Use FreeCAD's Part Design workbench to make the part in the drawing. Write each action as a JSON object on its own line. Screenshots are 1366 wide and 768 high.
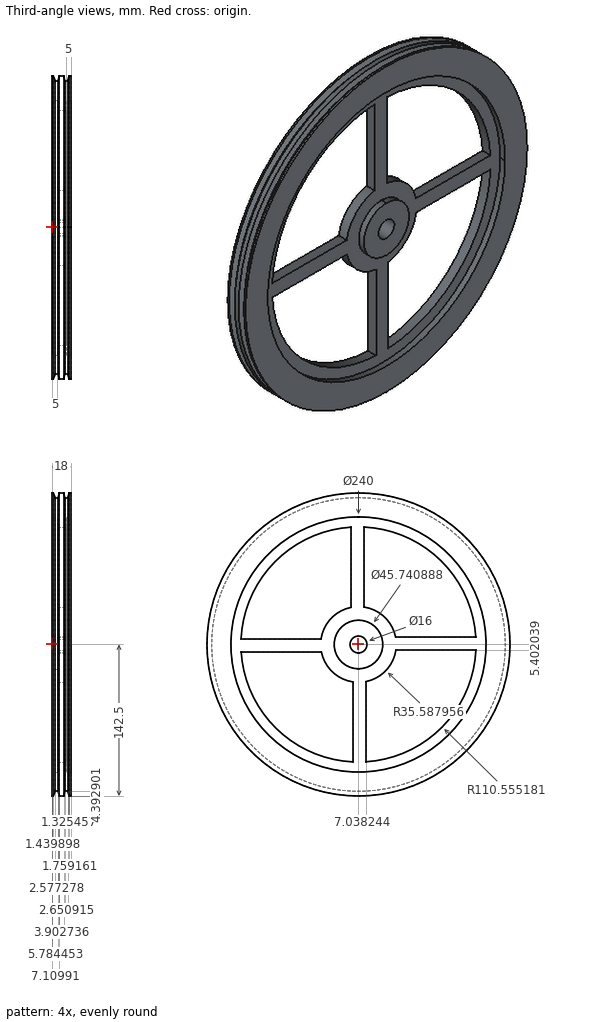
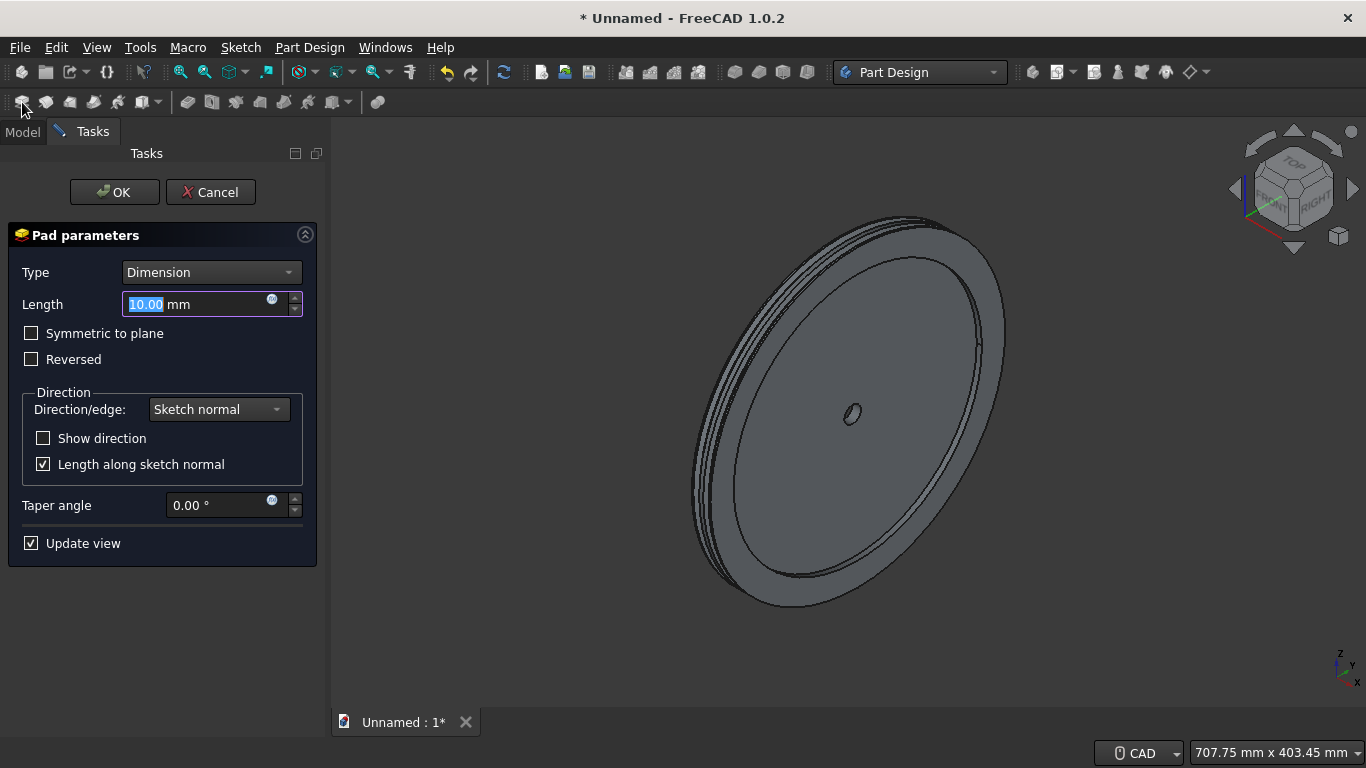
{"action": "type", "text": "5"}
{"action": "key", "text": "Tab"}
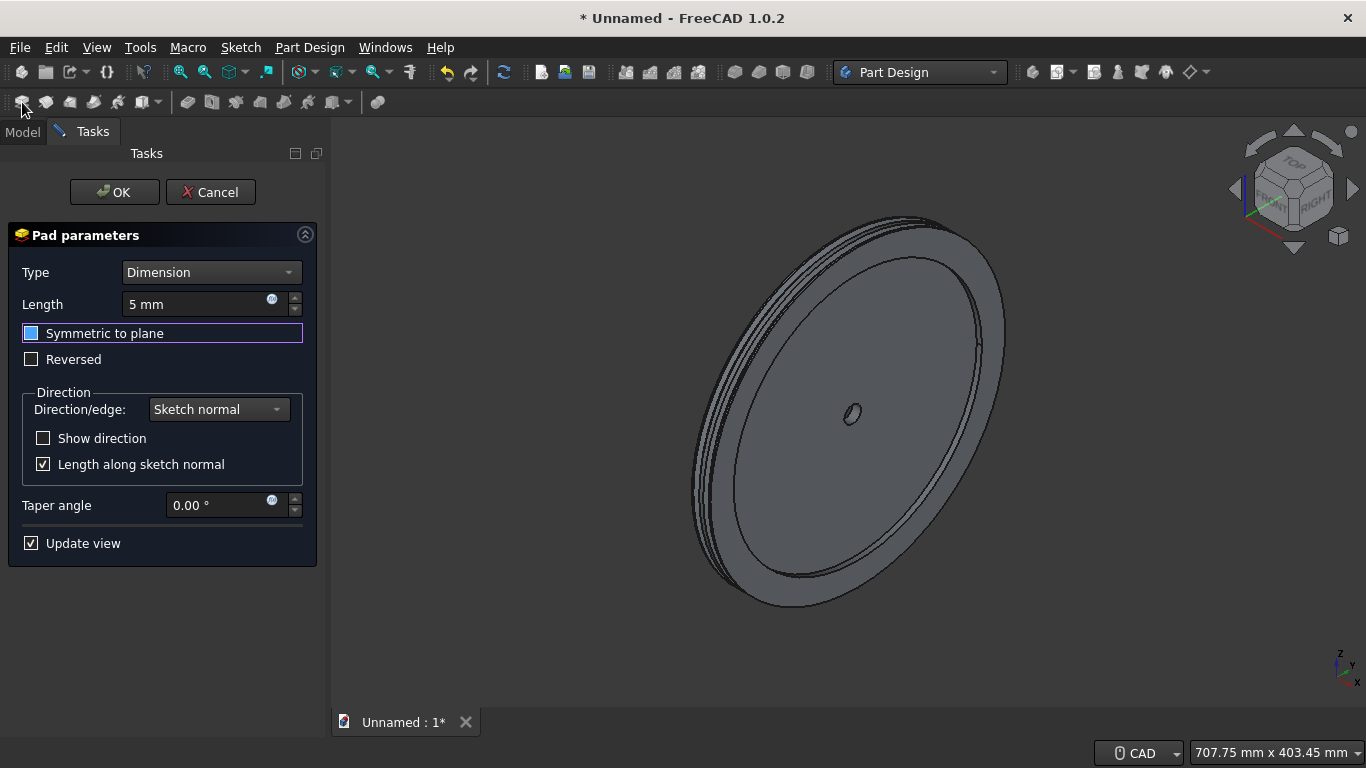
{"action": "left_click", "coordinate": [30, 359]}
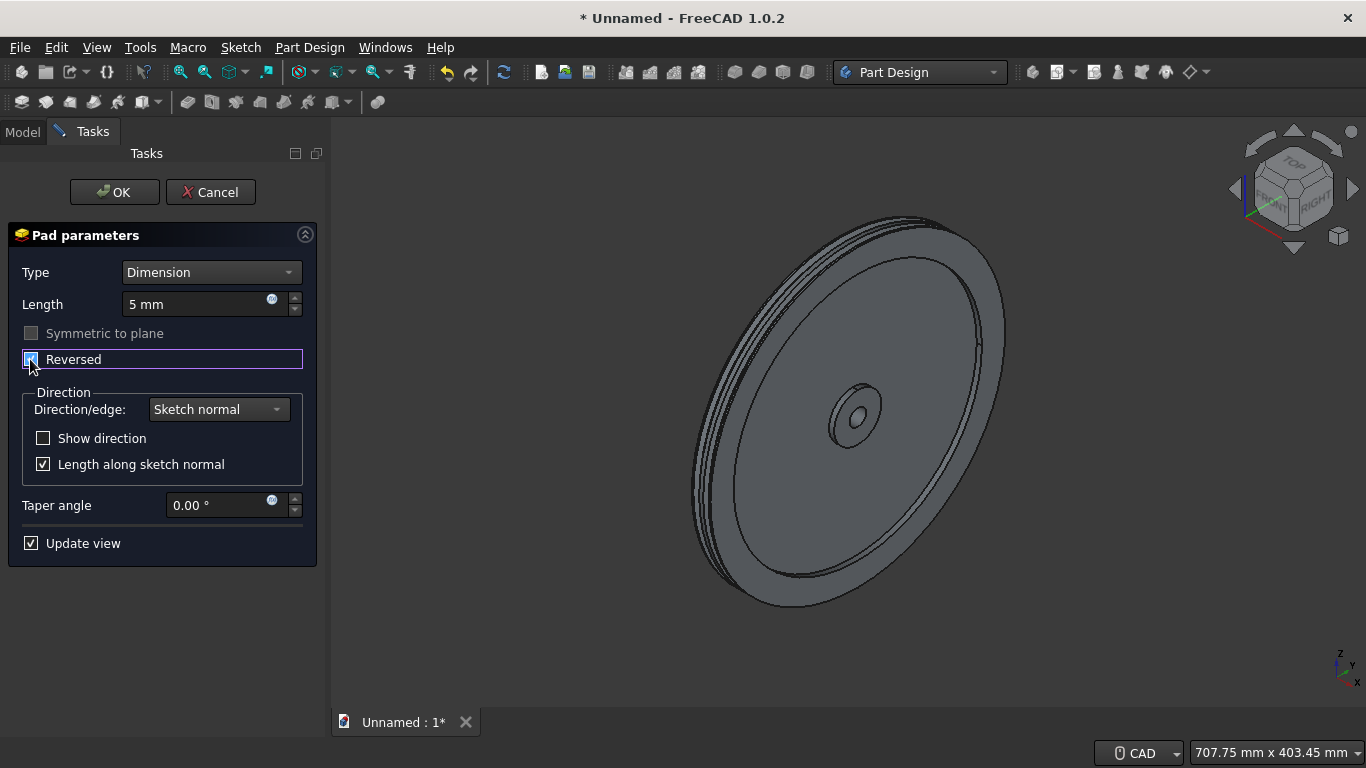
{"action": "left_click", "coordinate": [115, 192]}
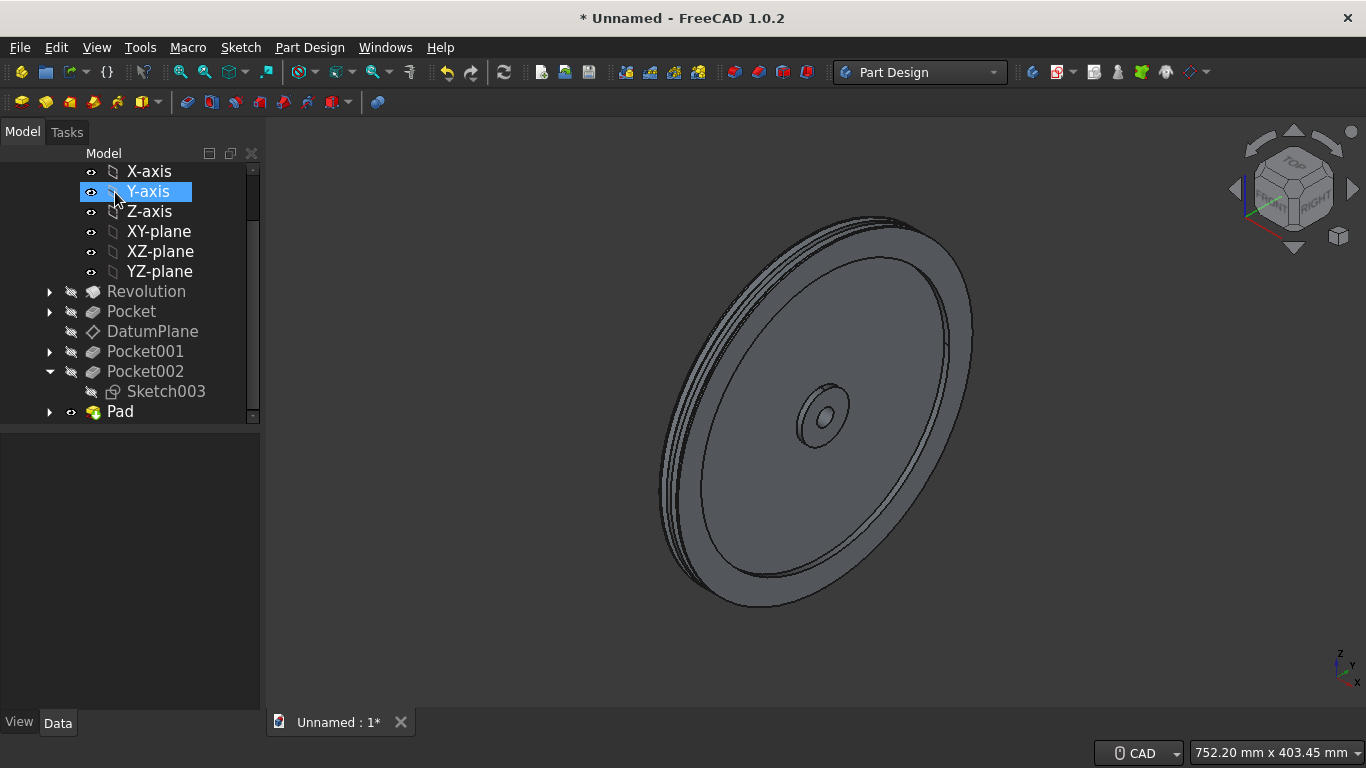
{"action": "key", "text": "6"}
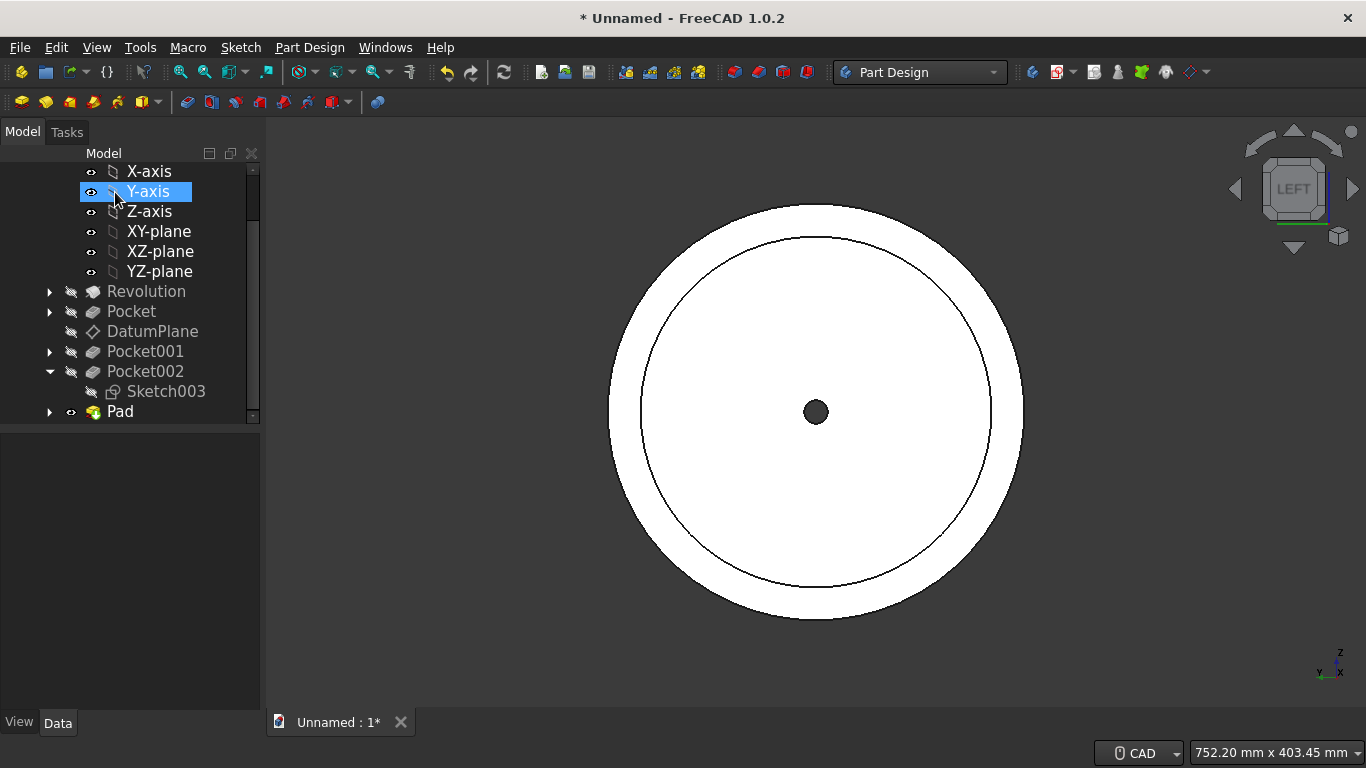
{"action": "left_click", "coordinate": [716, 411]}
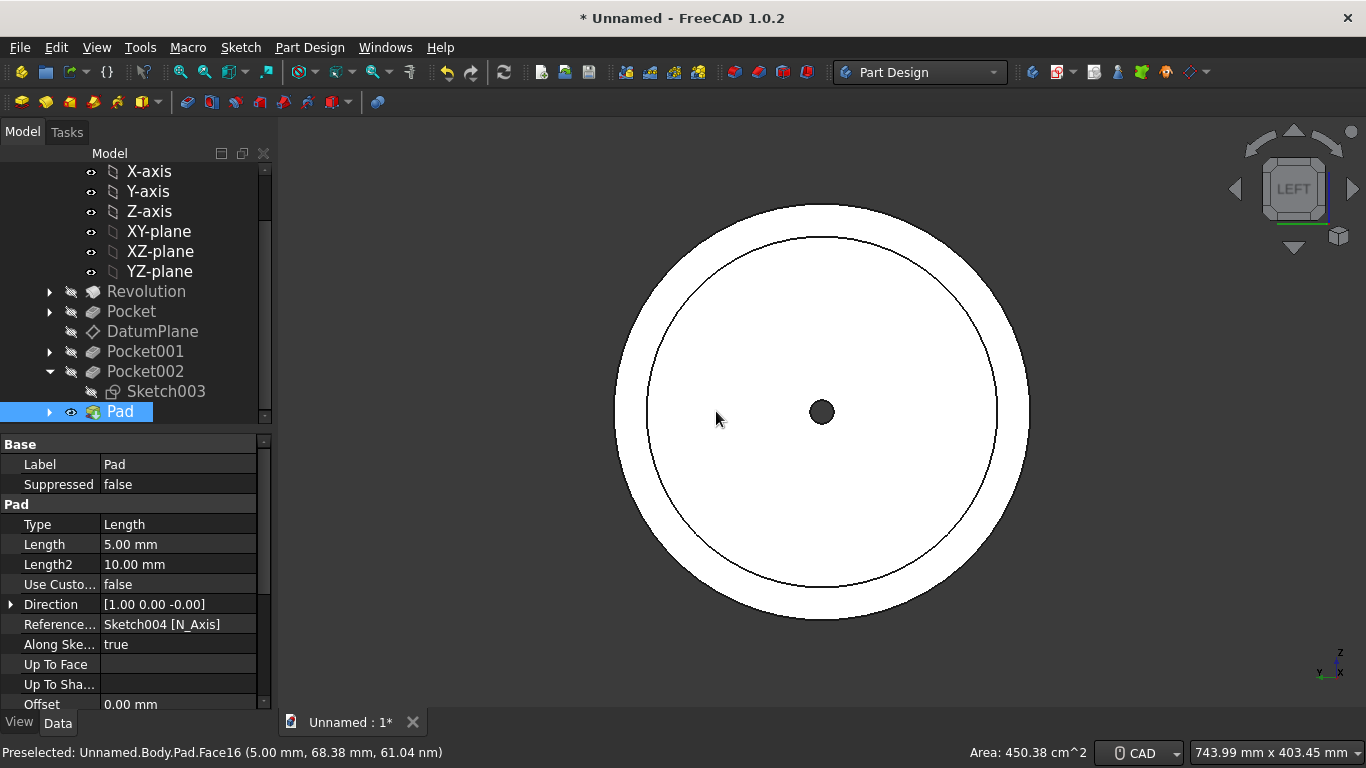
{"action": "left_click", "coordinate": [1058, 72]}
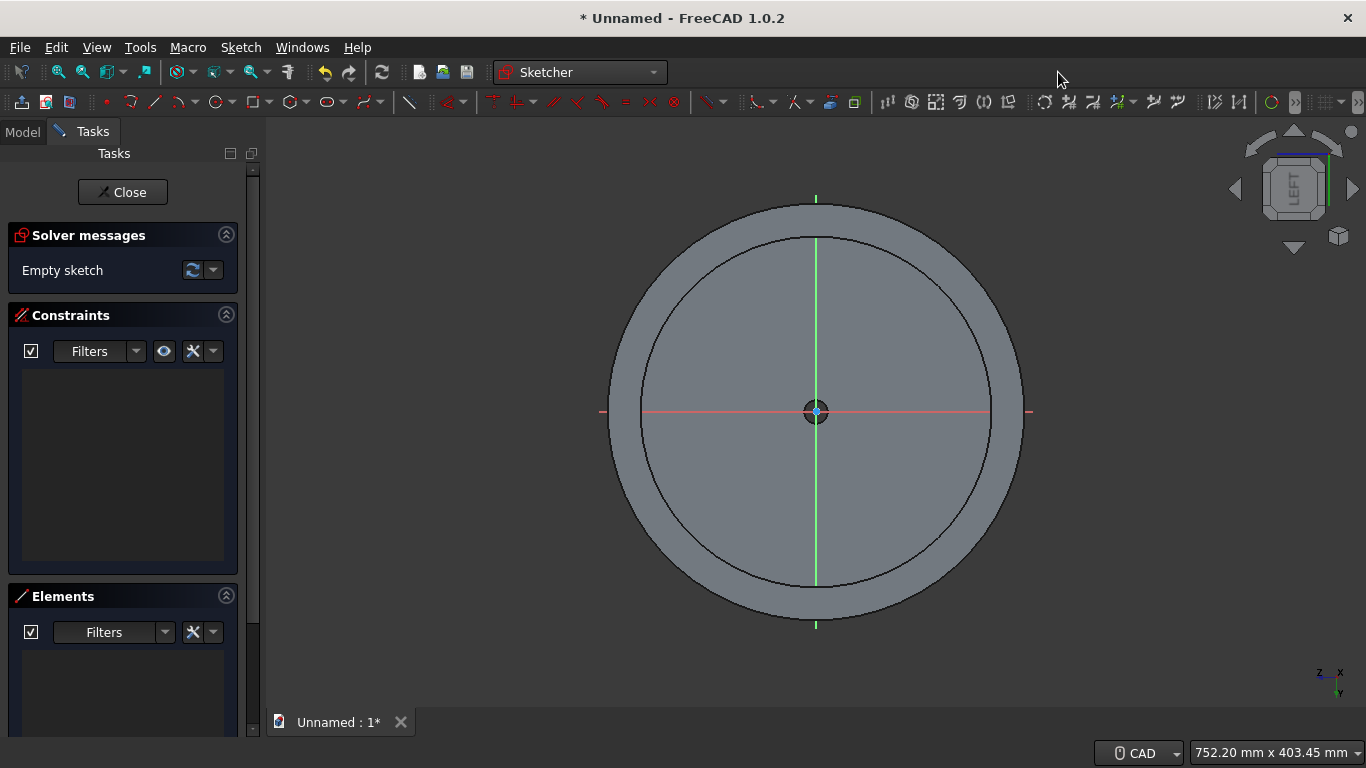
{"action": "key", "text": "q s"}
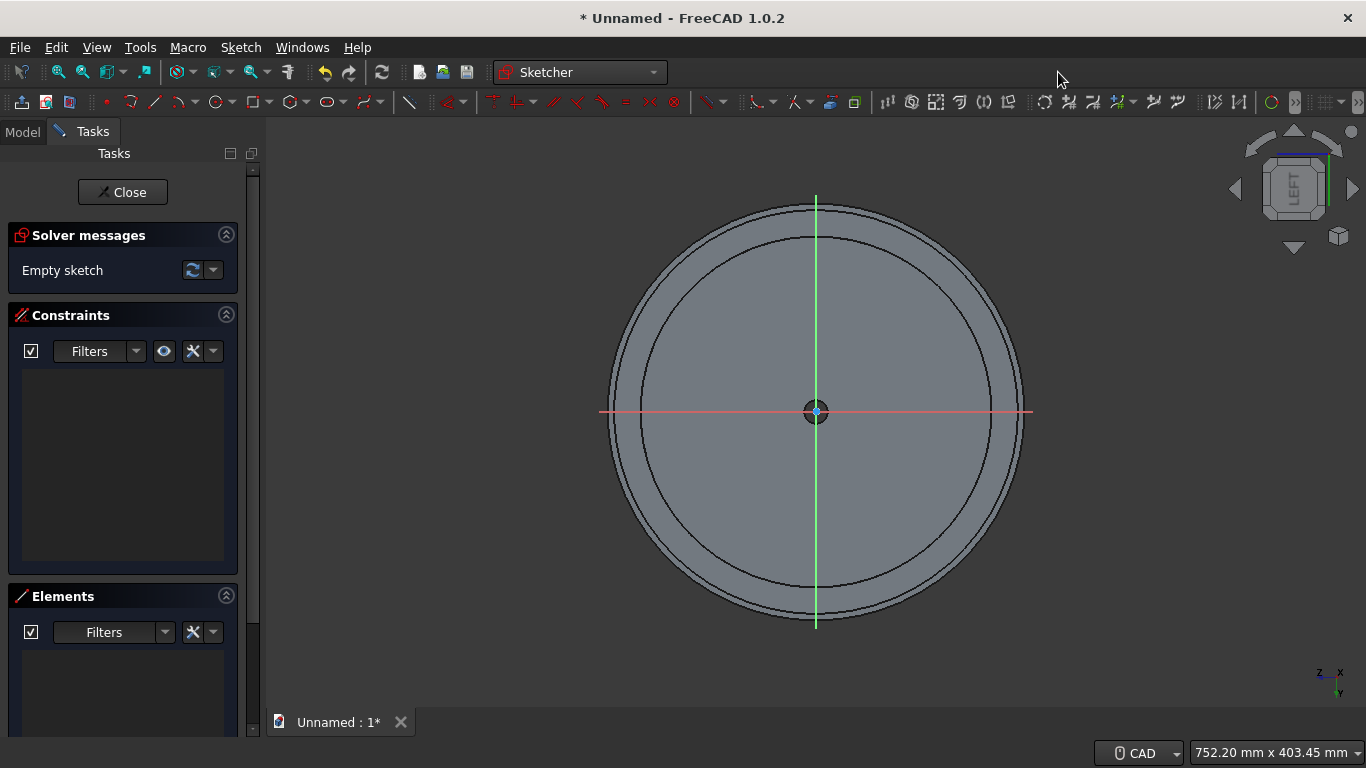
{"action": "scroll", "coordinate": [830, 412], "scroll_direction": "up", "scroll_amount": 9}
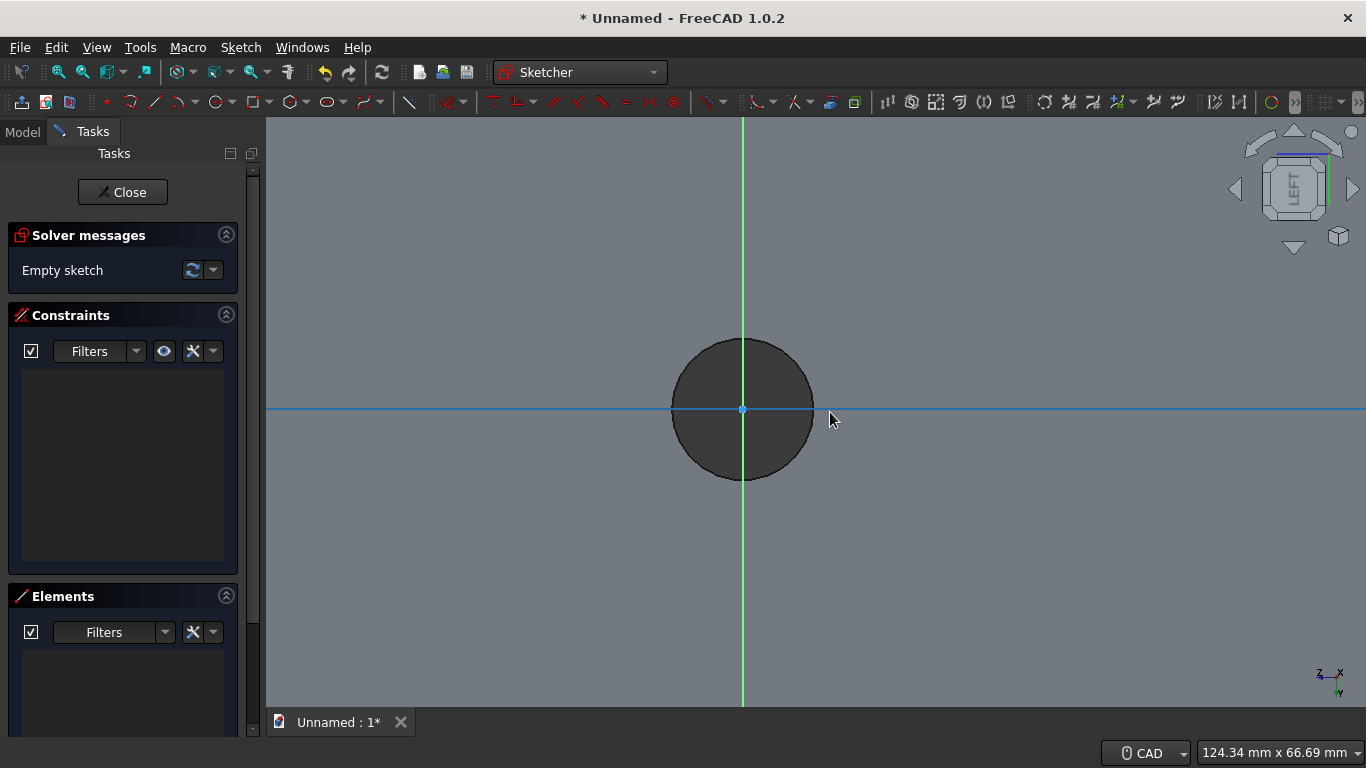
{"action": "key", "text": "g c"}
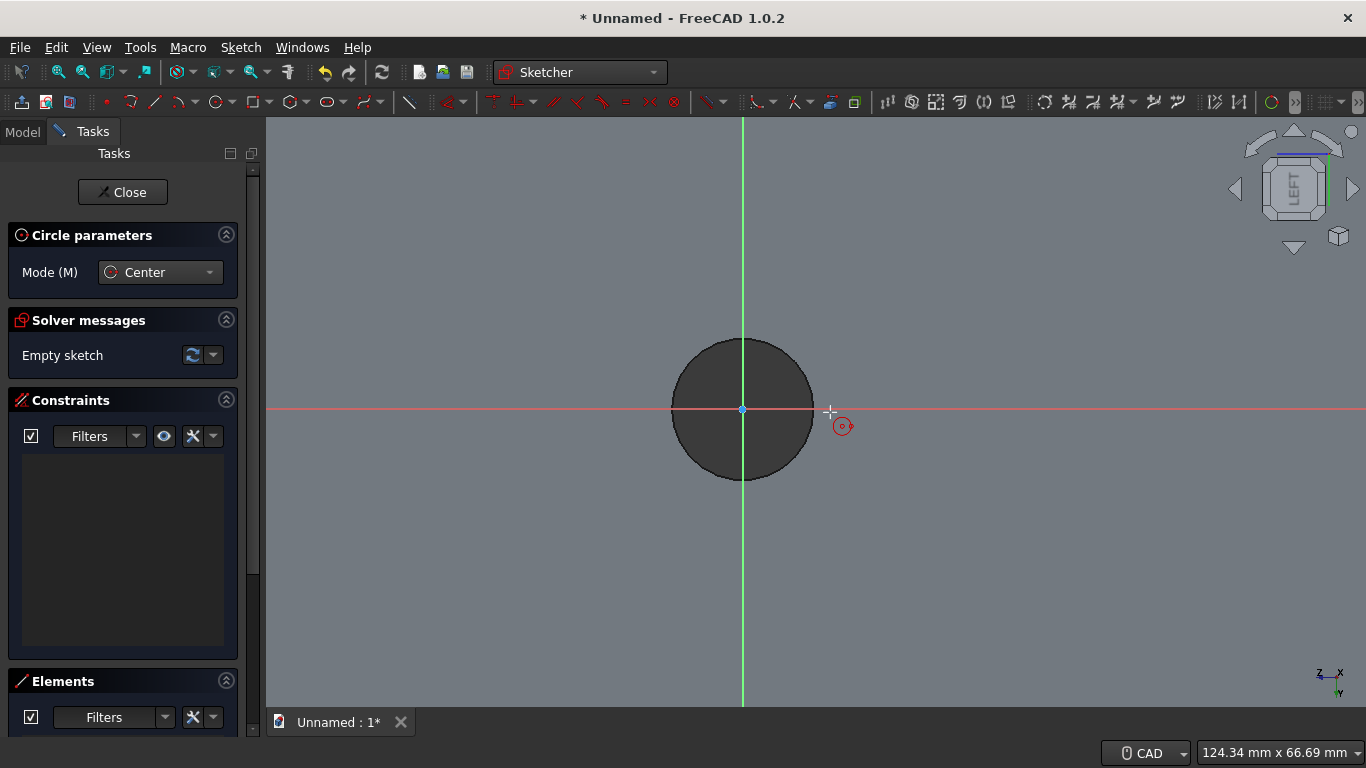
{"action": "left_click", "coordinate": [743, 409]}
{"action": "mouse_move", "coordinate": [886, 266]}